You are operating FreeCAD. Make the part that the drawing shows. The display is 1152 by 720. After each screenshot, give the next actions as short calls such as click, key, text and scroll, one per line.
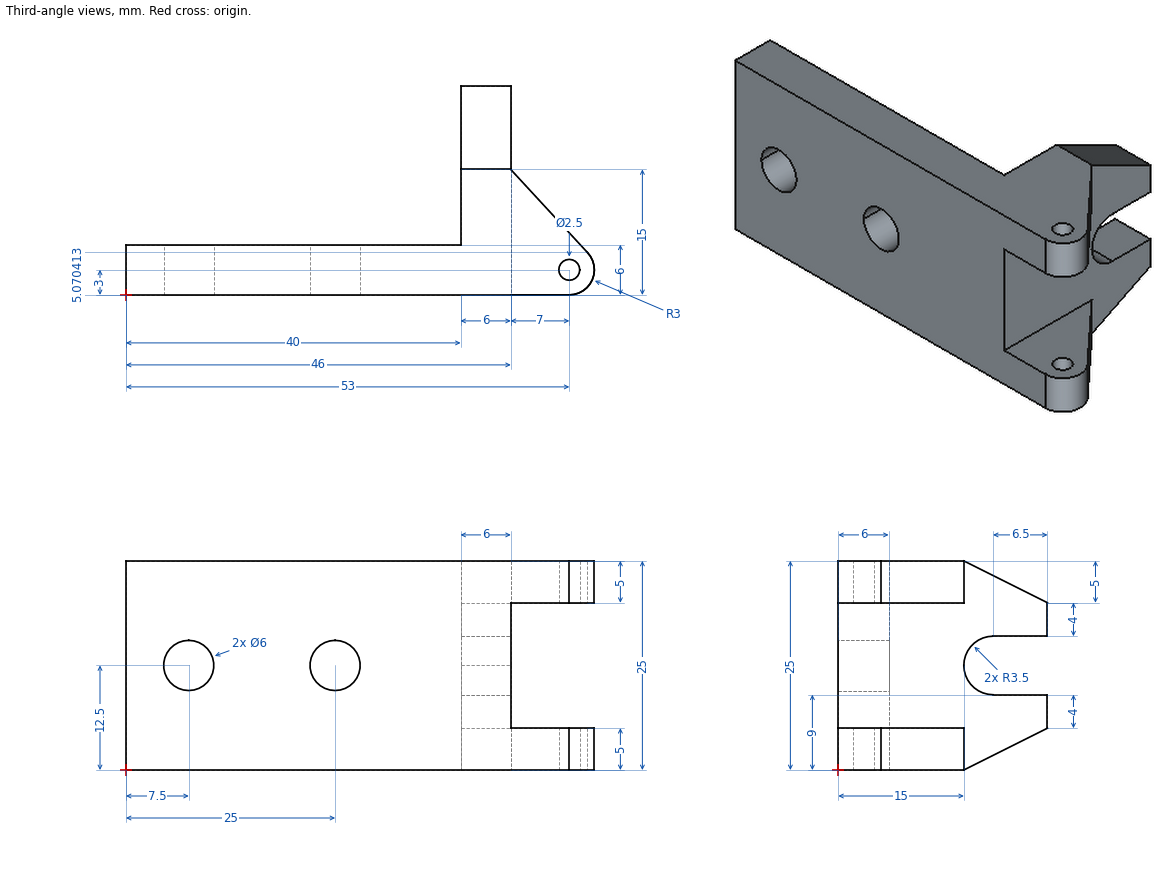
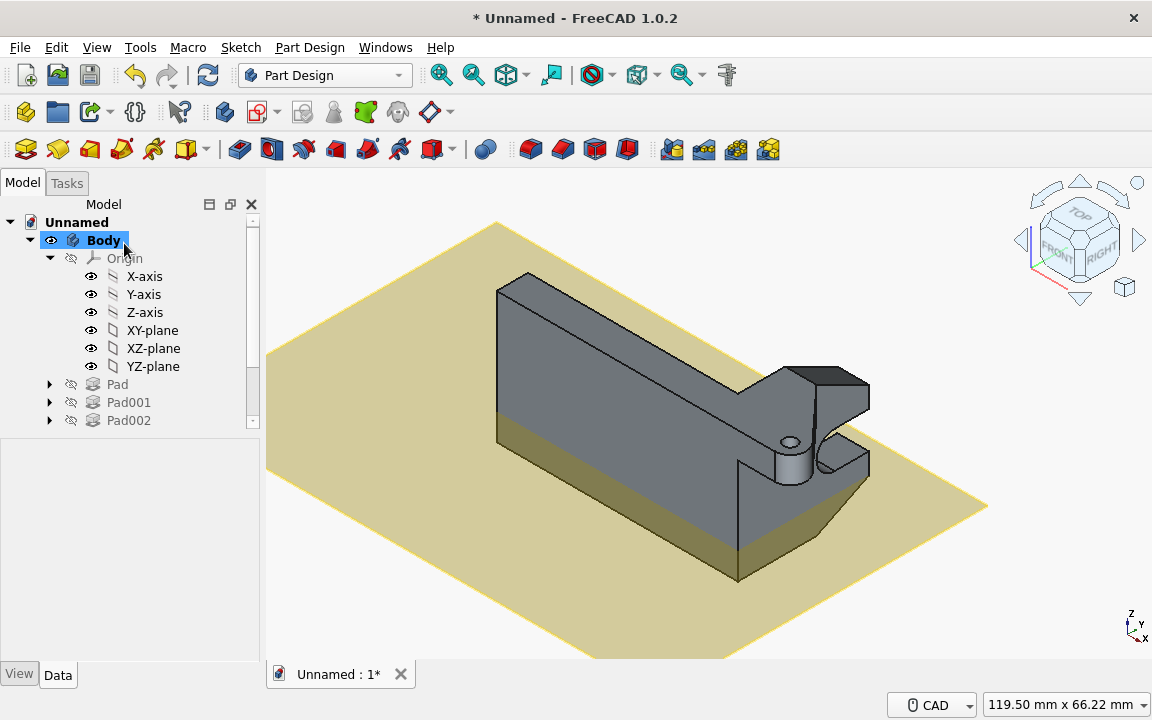
scroll(100, 326, down, 3)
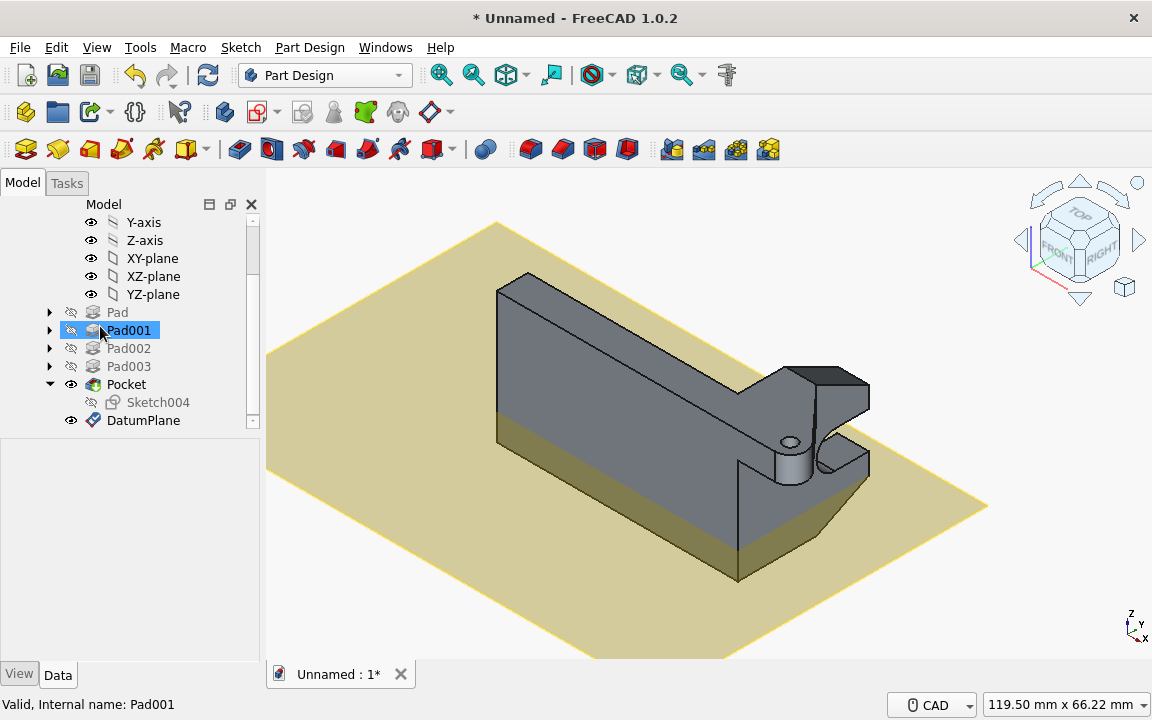
click(116, 420)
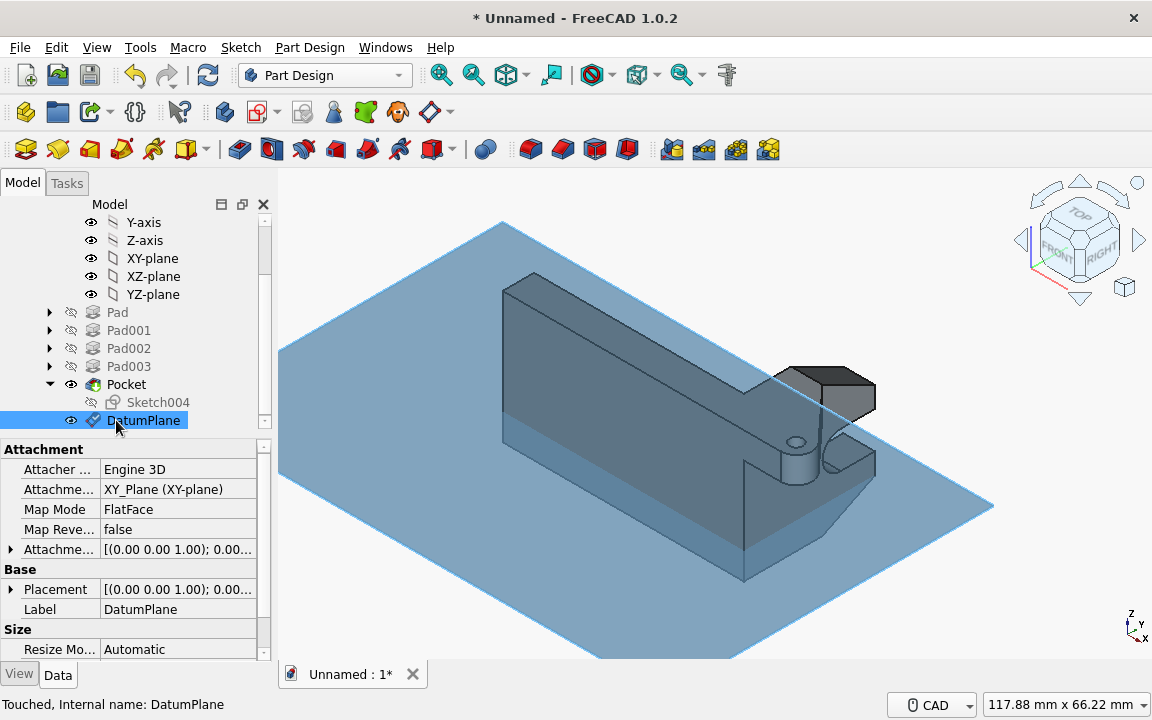
click(258, 112)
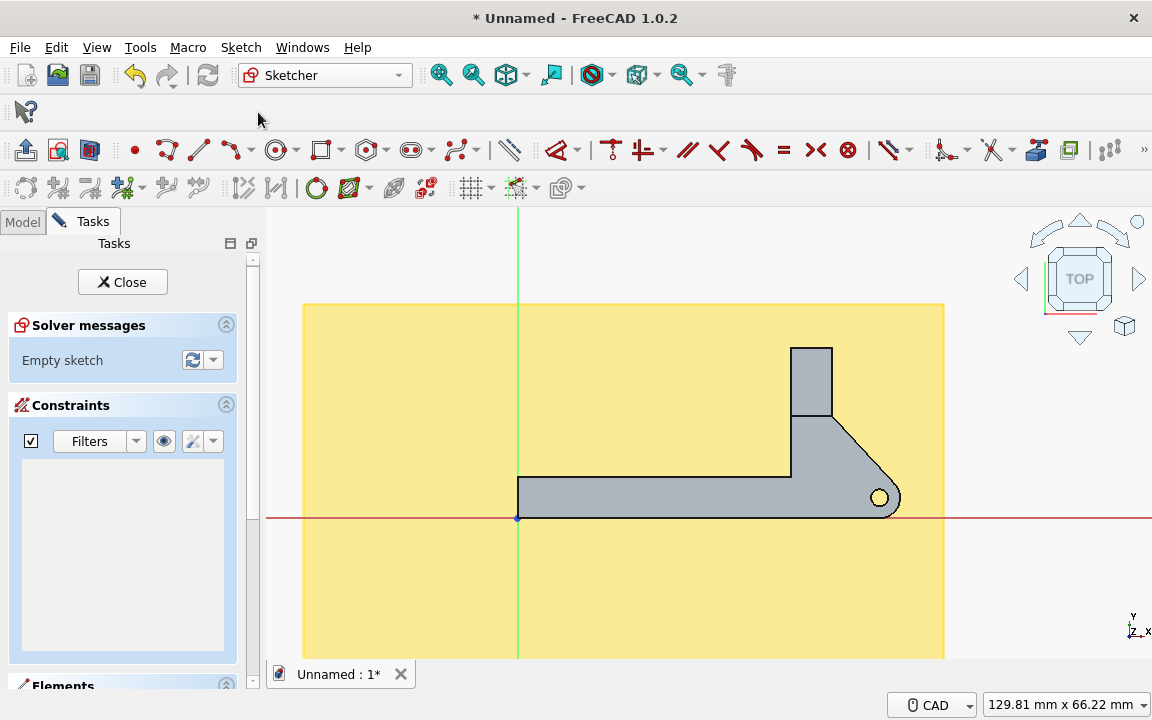
click(90, 150)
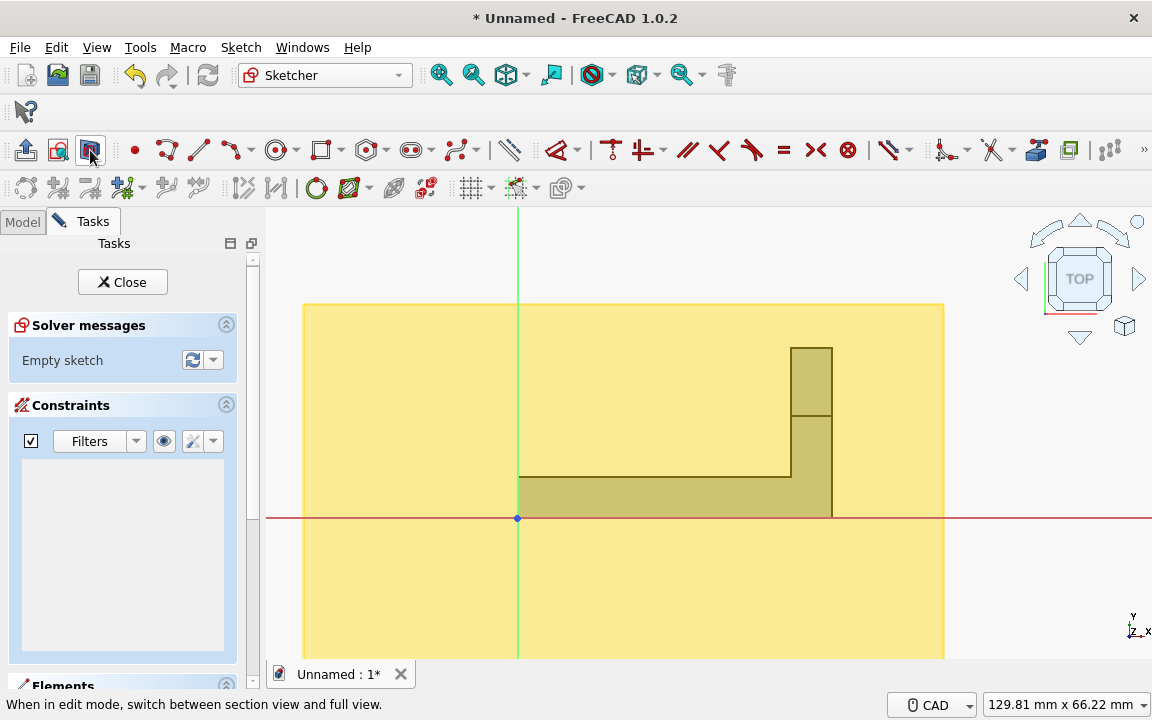
scroll(987, 487, up, 5)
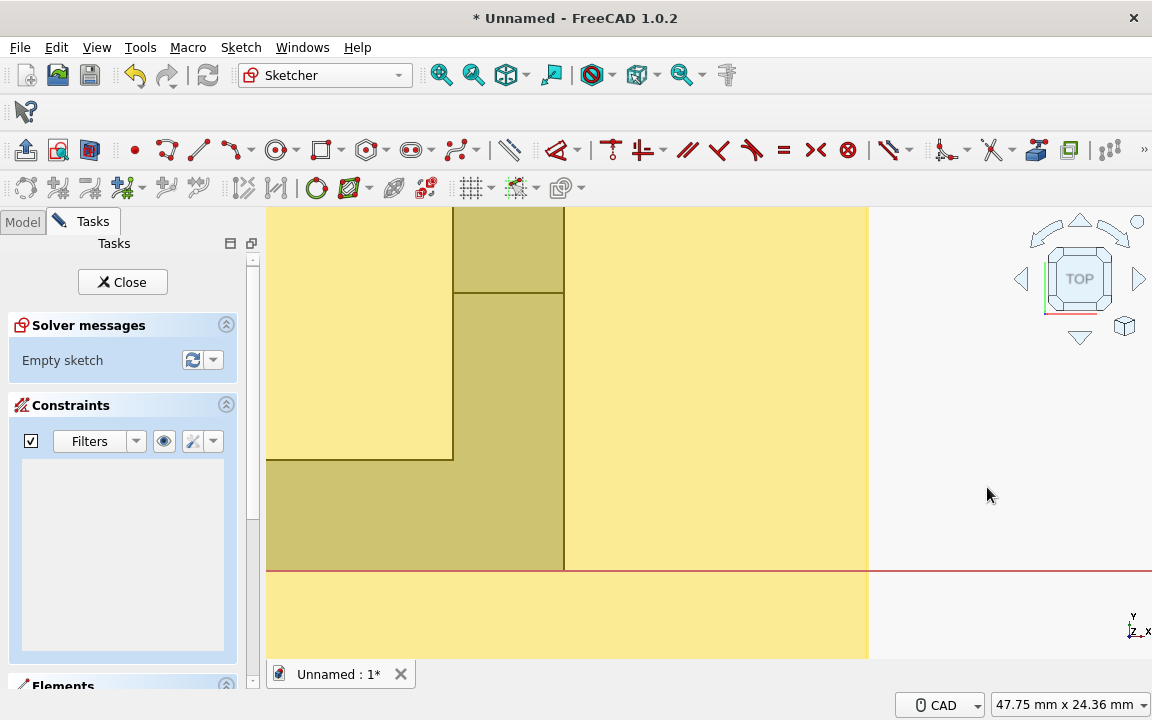
key(g)
key(m)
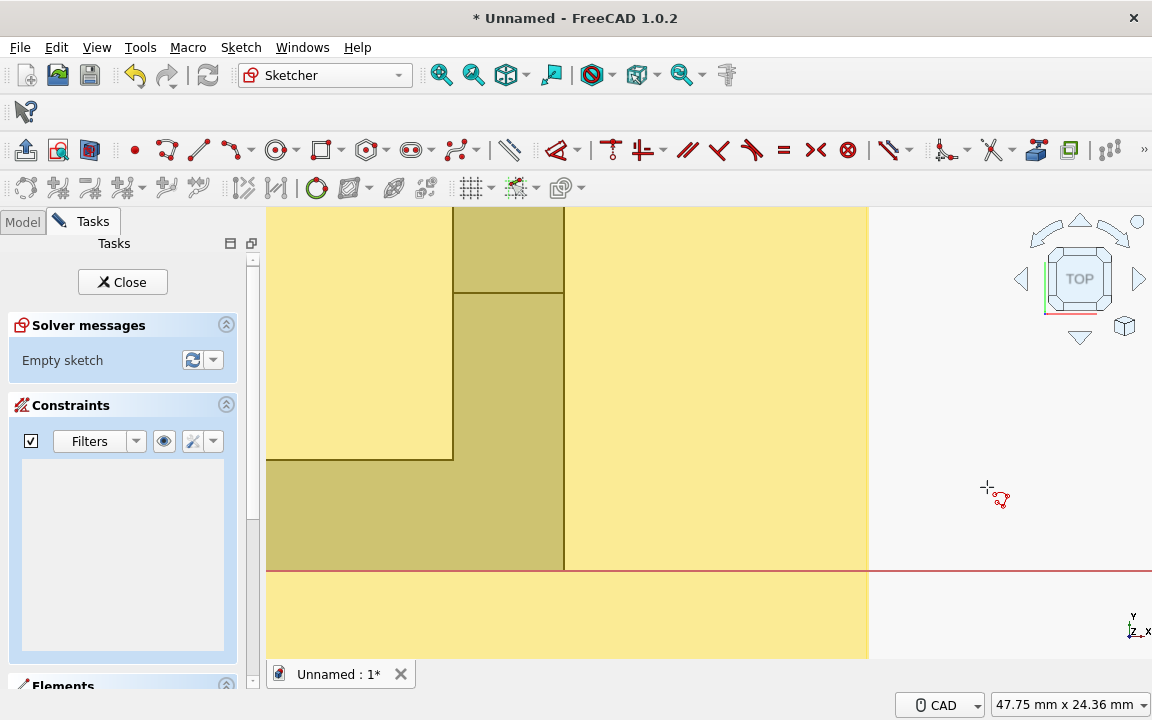
click(694, 571)
click(564, 562)
click(564, 293)
click(734, 477)
right_click(734, 477)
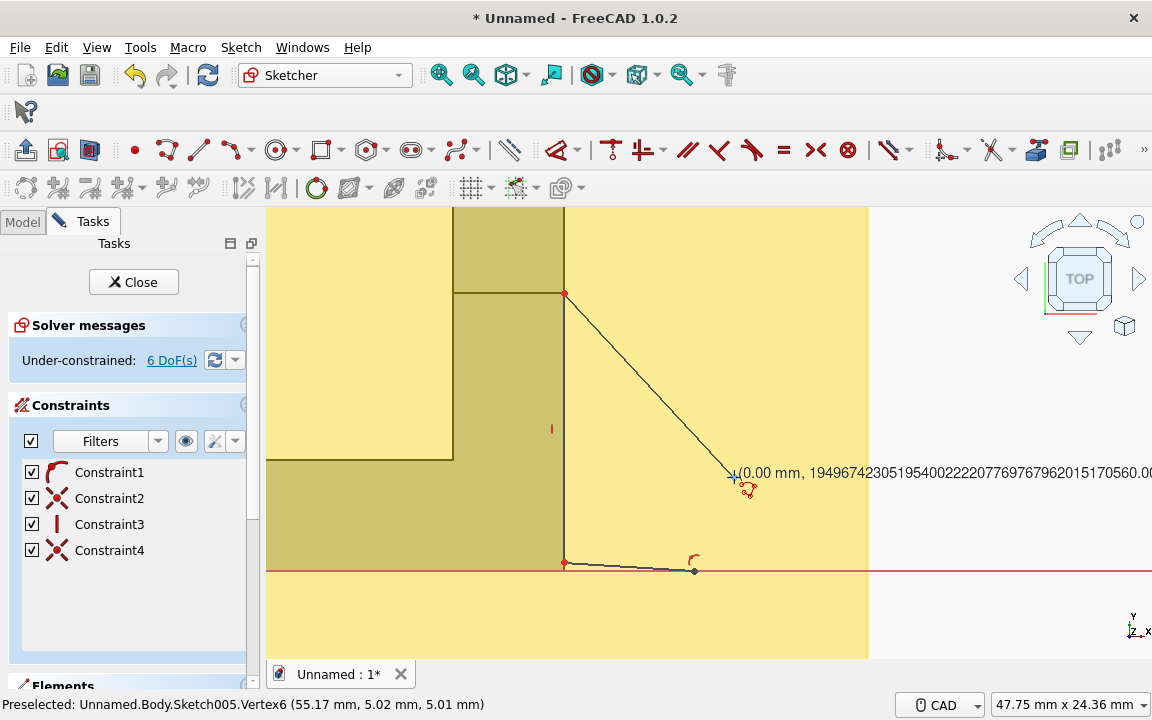
key(g)
key(3)
key(a)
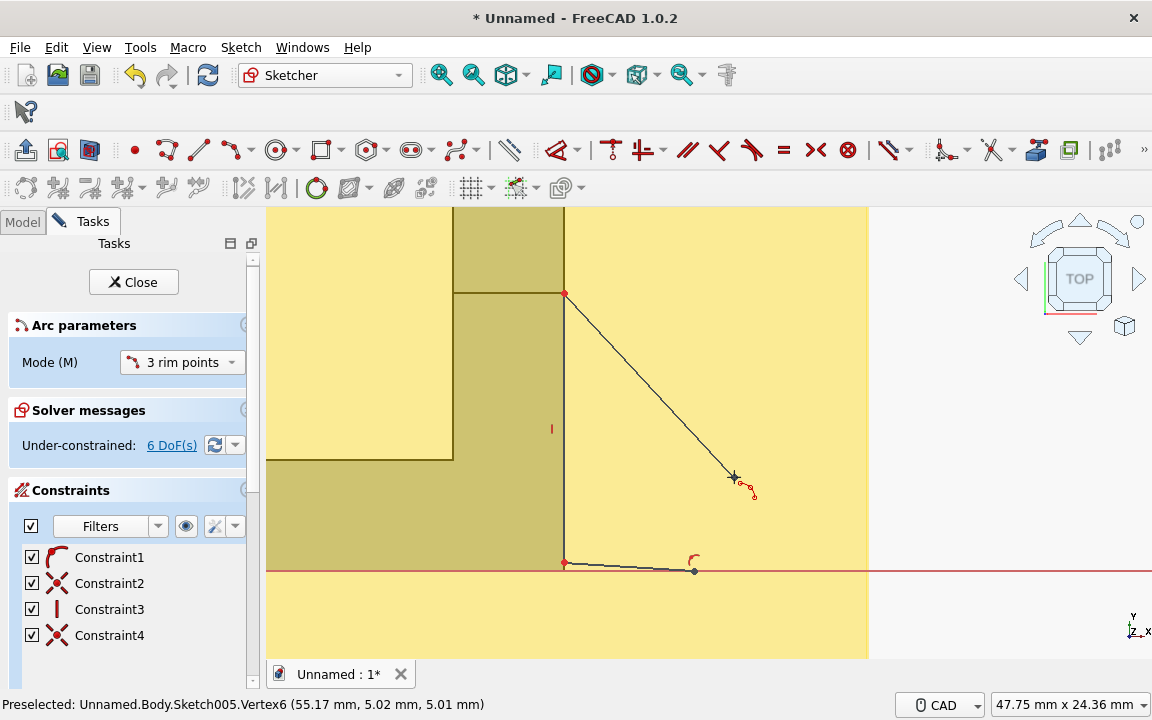
click(734, 478)
click(694, 571)
click(745, 537)
key(Escape)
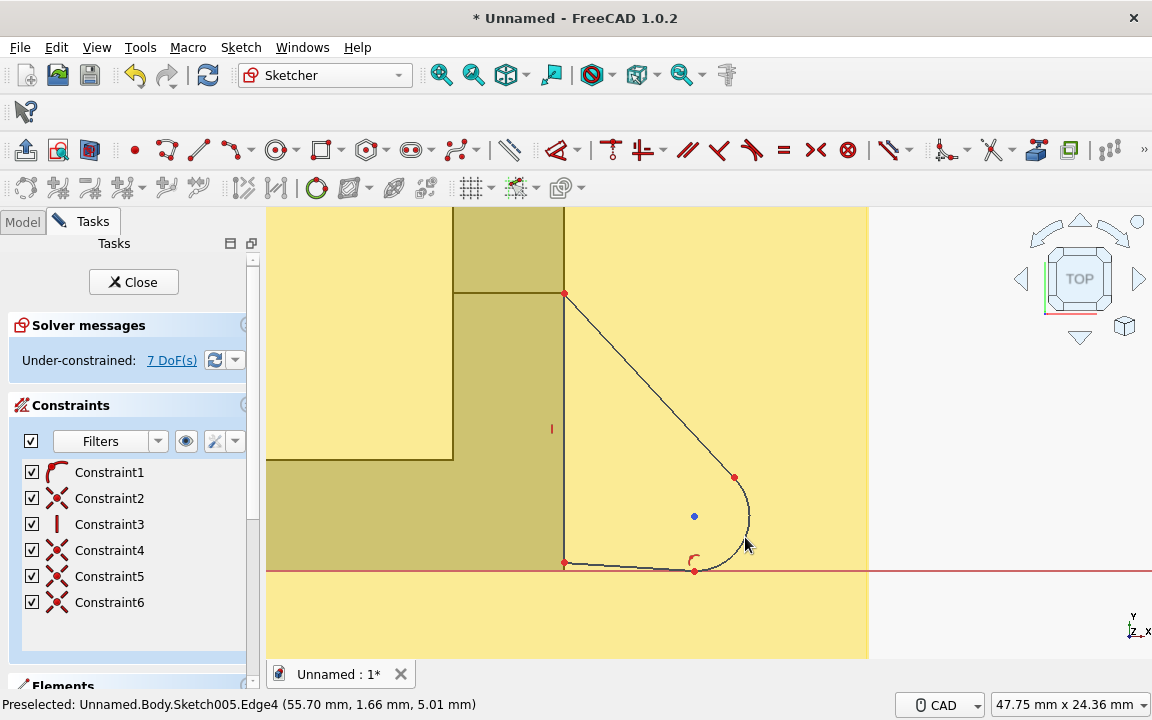
click(655, 569)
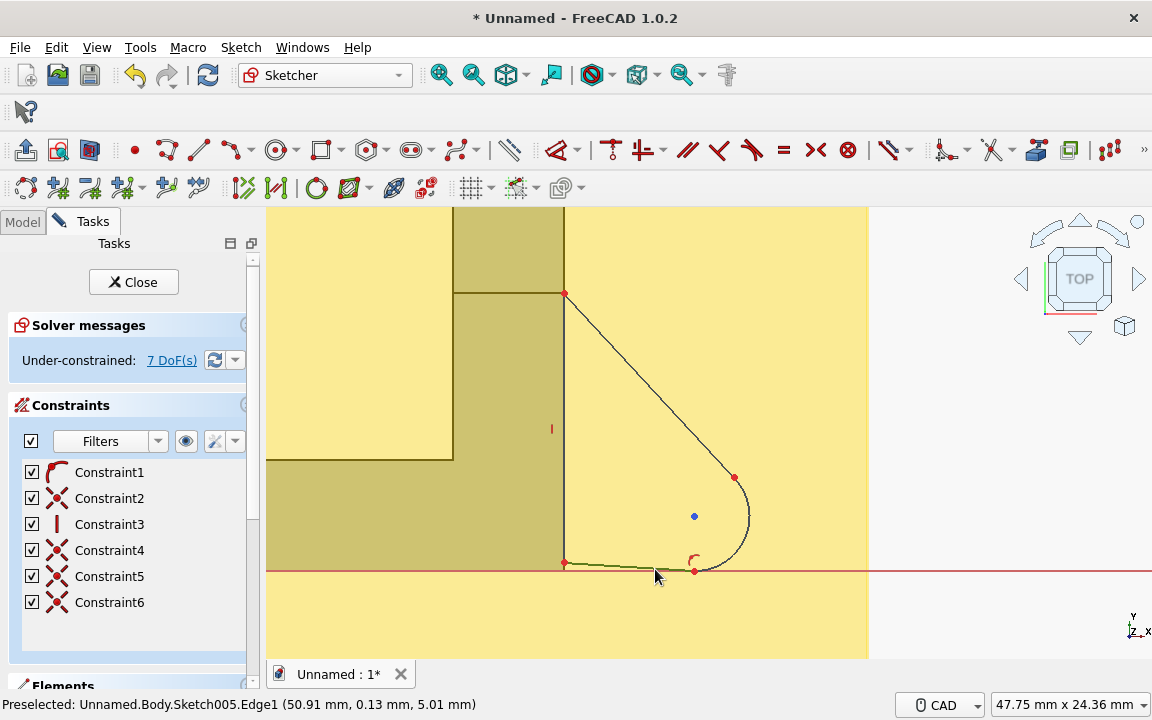
click(730, 558)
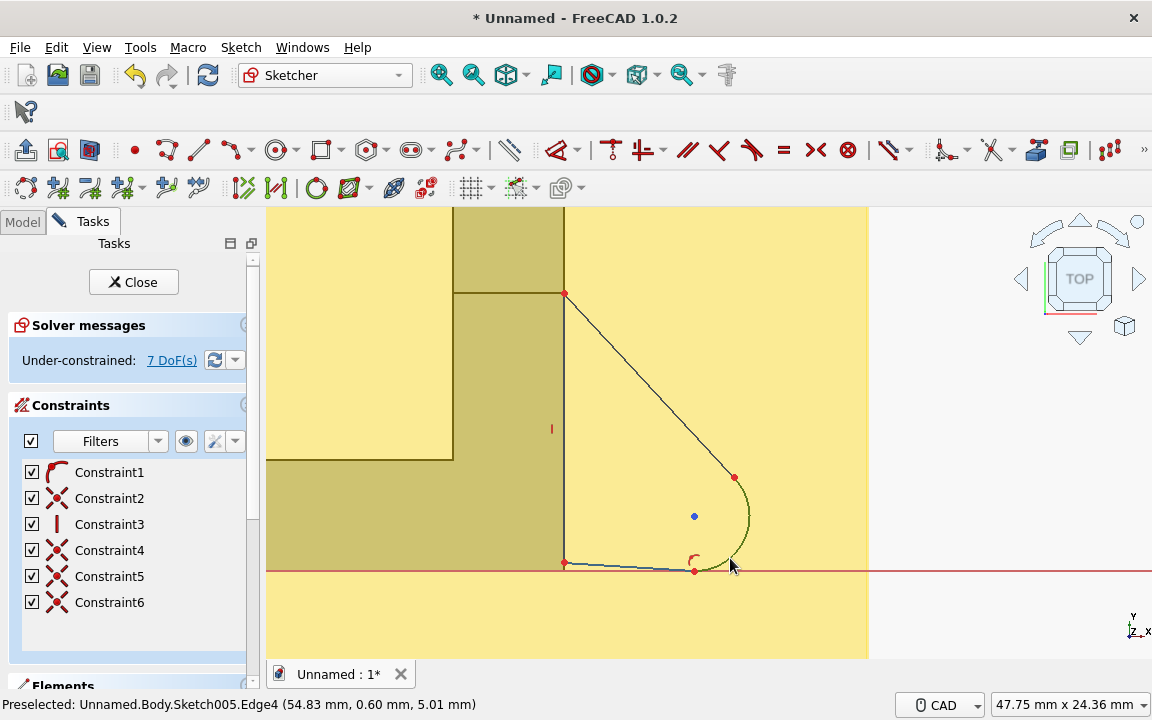
click(752, 150)